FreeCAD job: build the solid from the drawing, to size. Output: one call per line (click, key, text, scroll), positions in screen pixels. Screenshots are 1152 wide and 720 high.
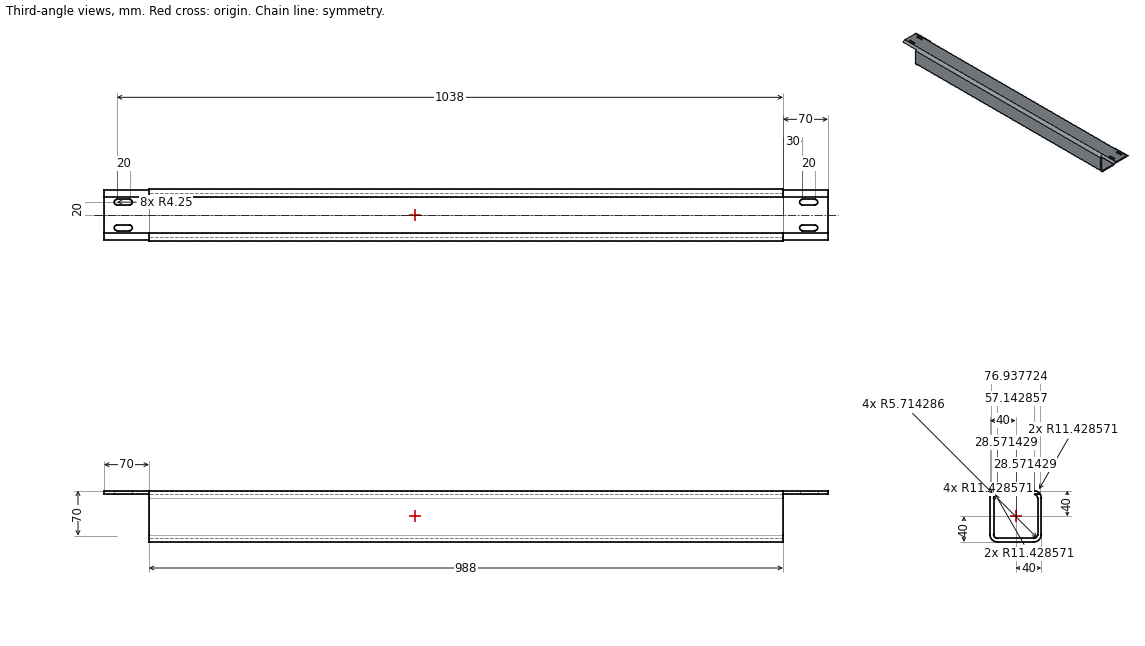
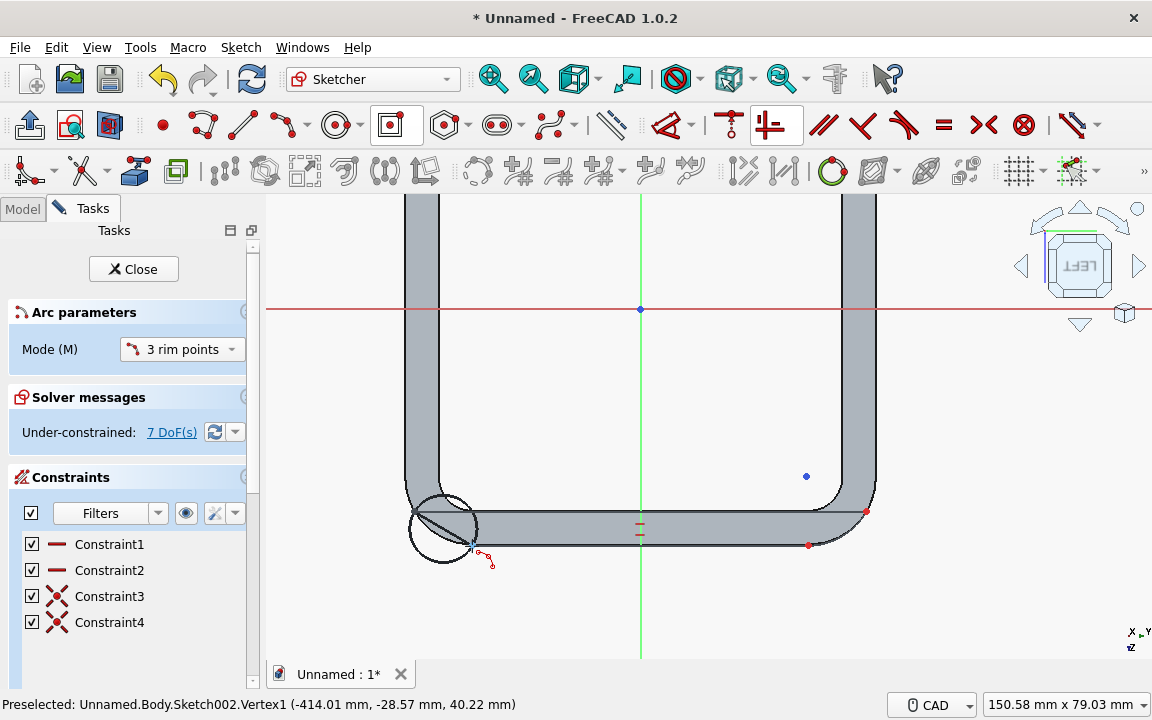
scroll(439, 536, up, 3)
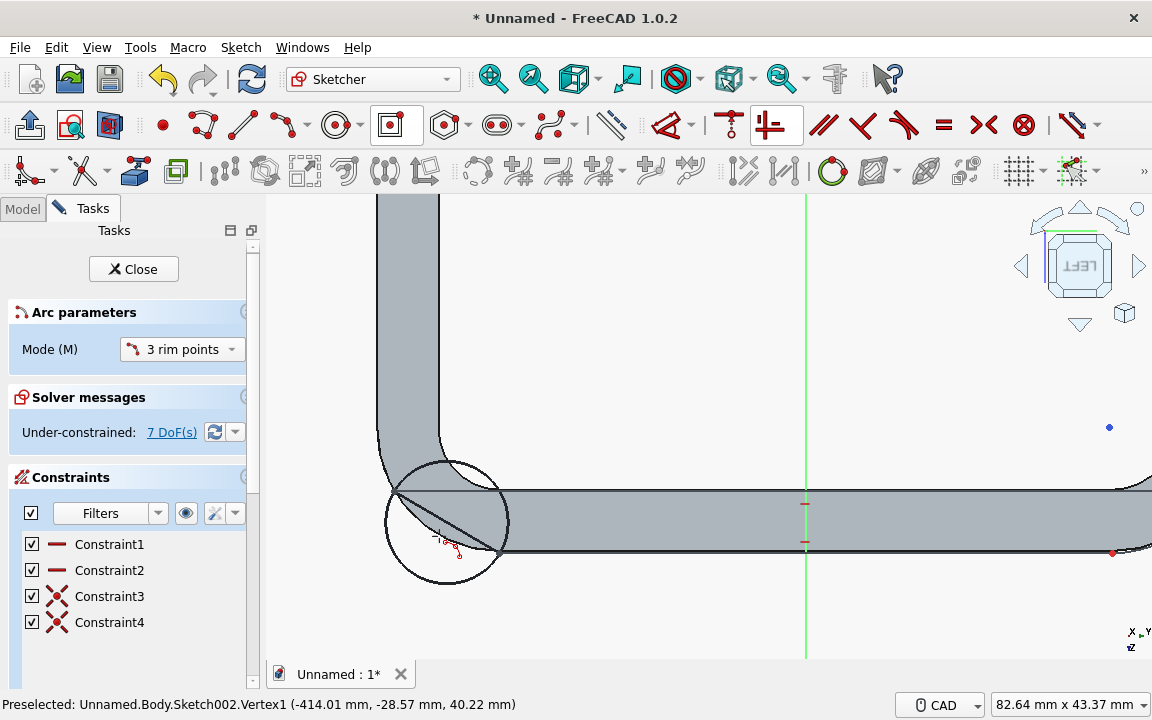
click(439, 535)
key(Escape)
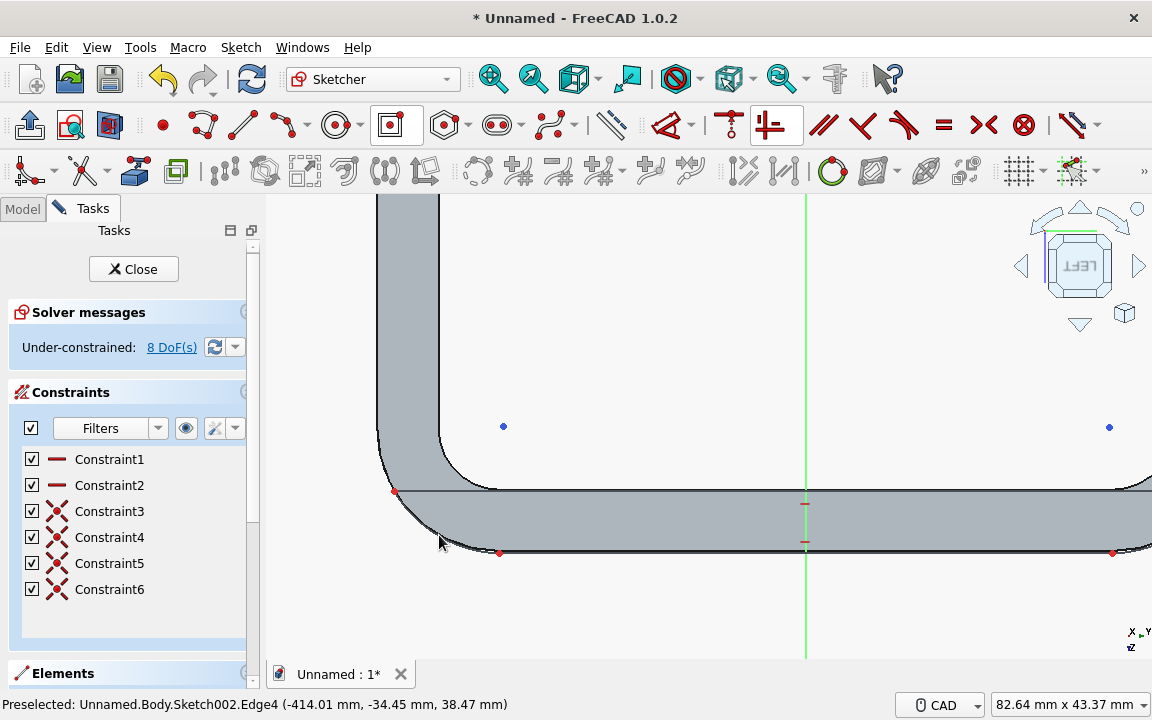
click(683, 553)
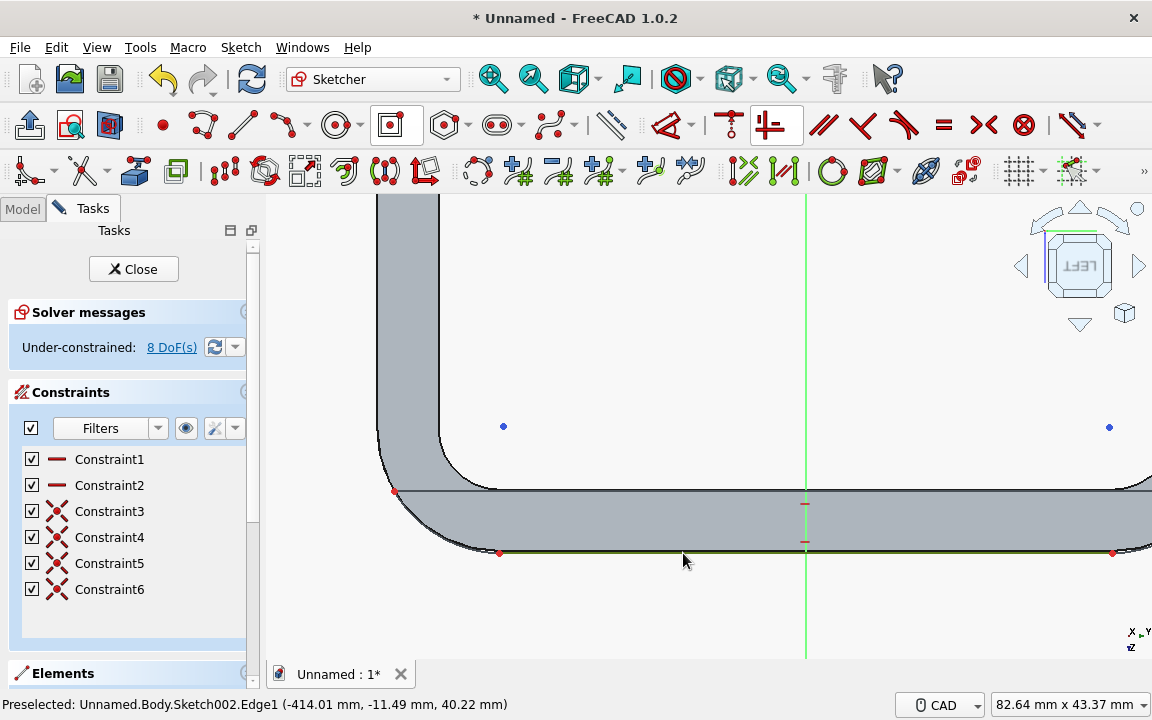
scroll(439, 536, down, 3)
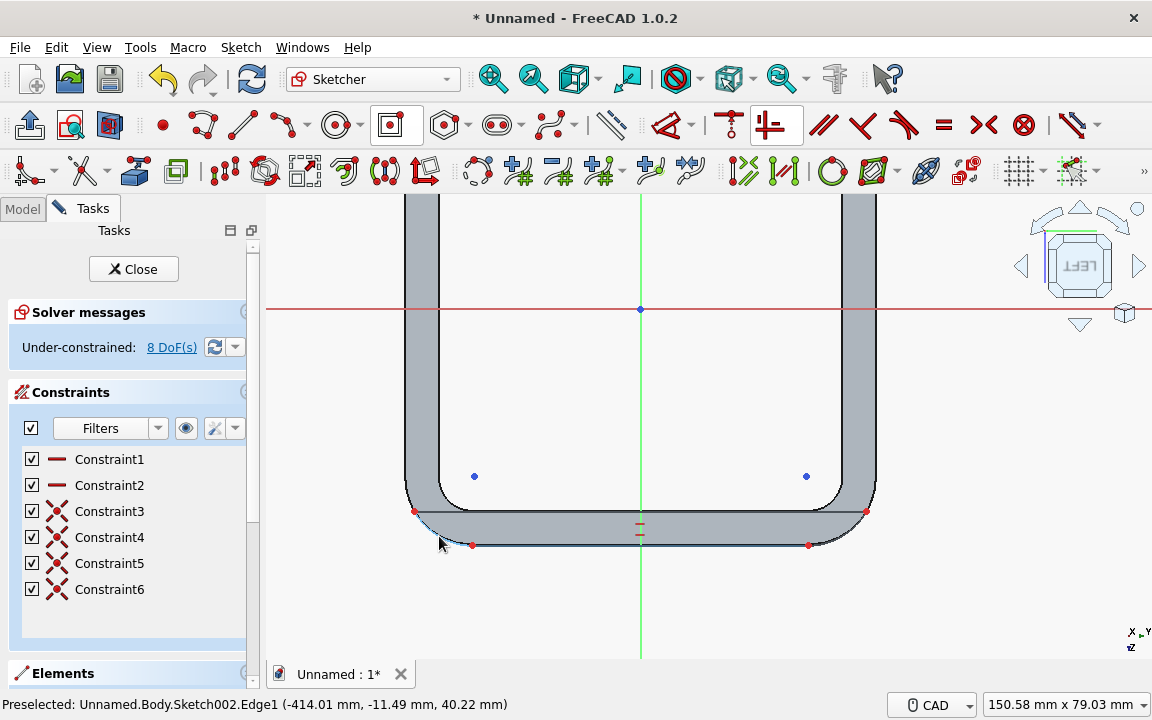
click(829, 542)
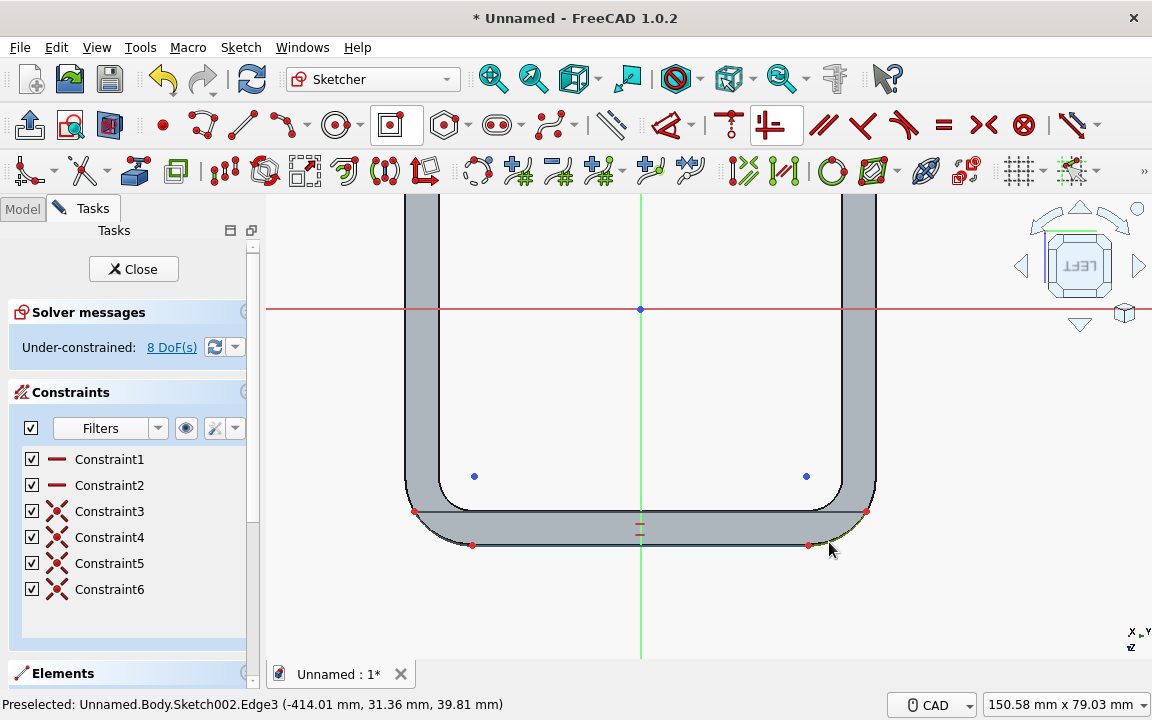
key(t)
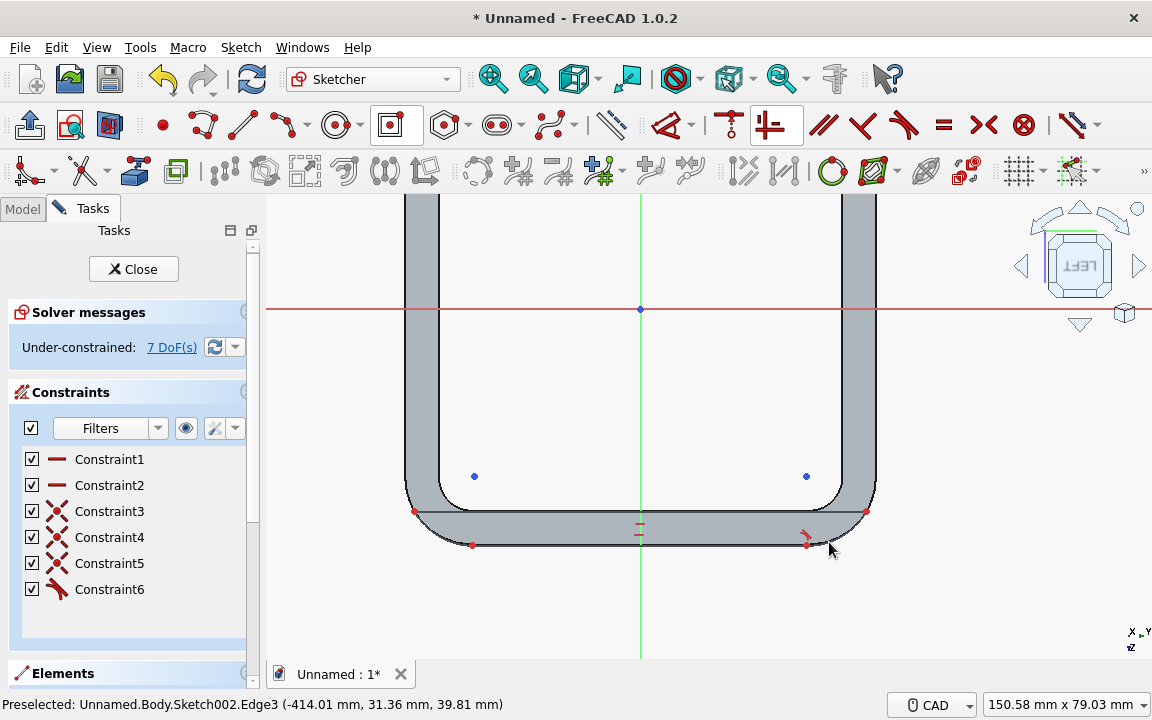
click(573, 546)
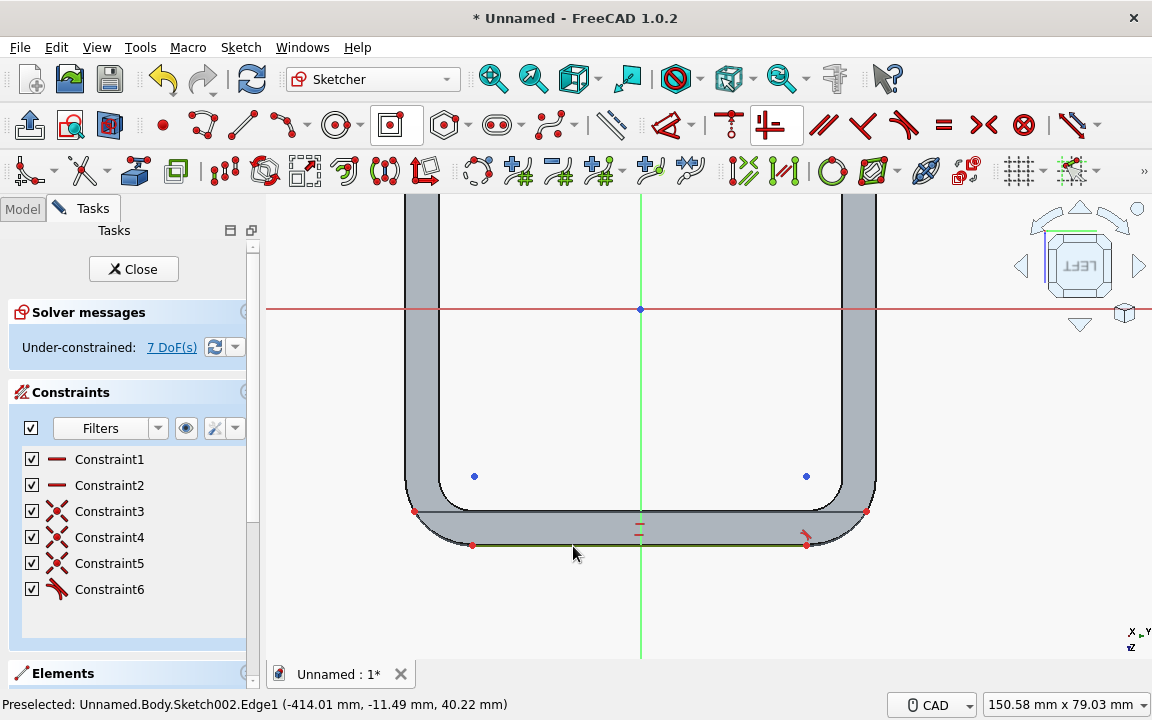
click(428, 528)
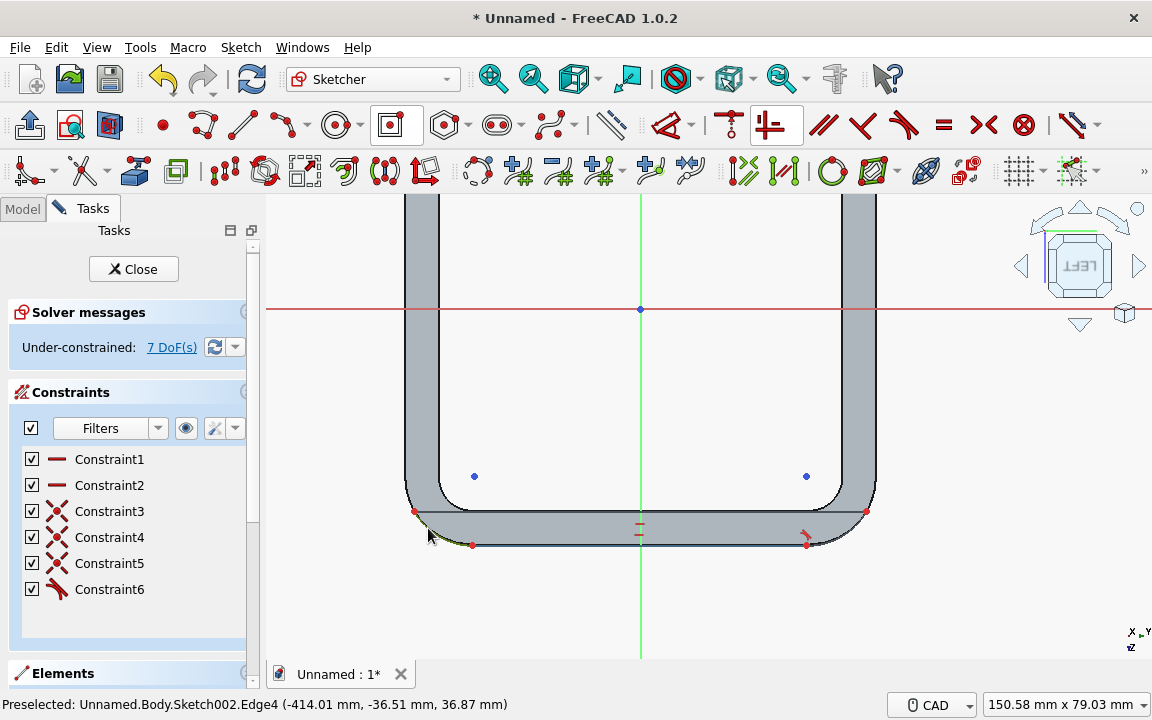
key(t)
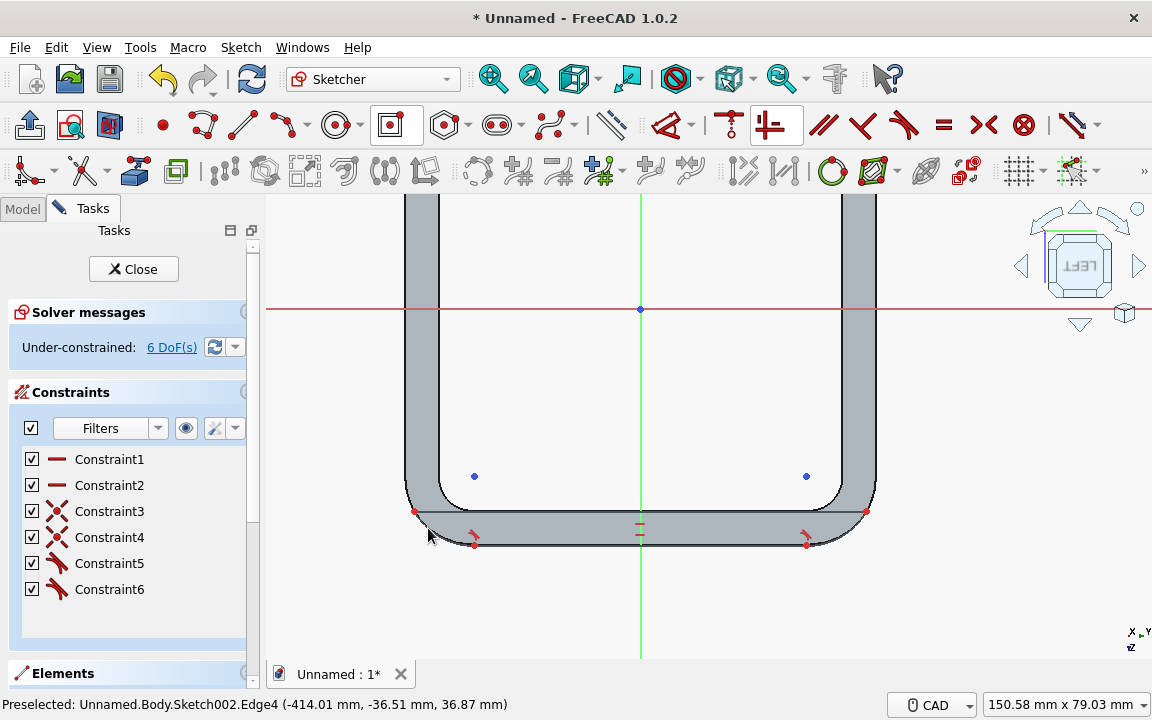
click(828, 543)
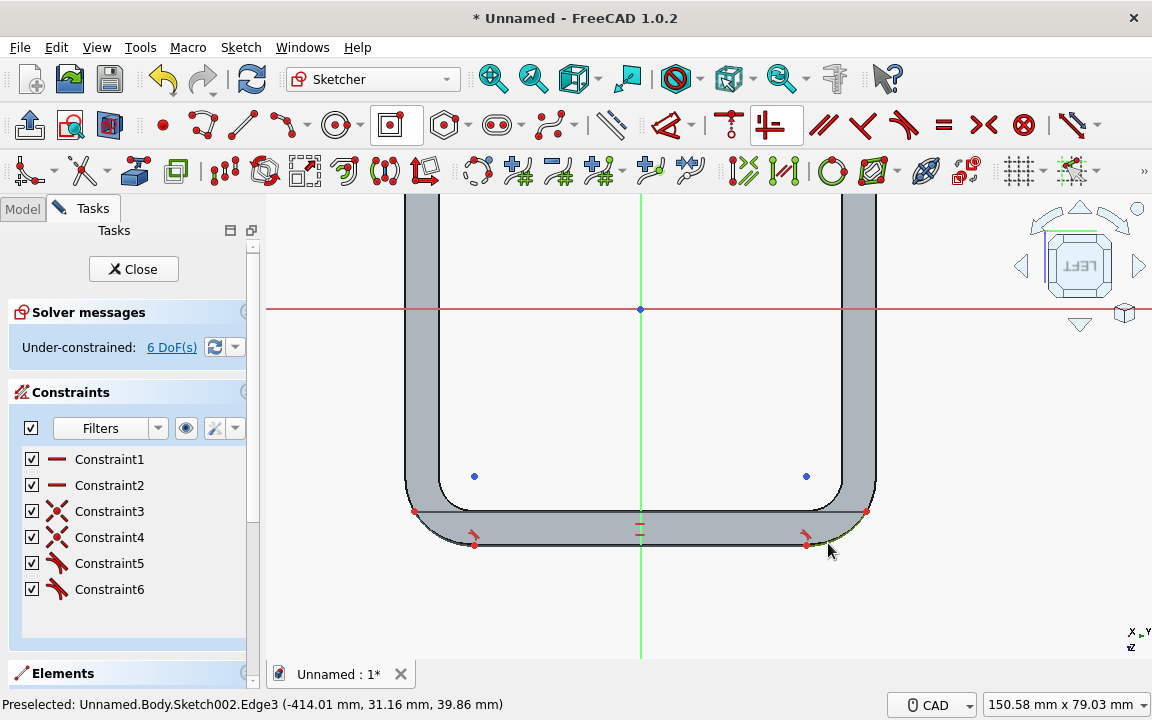
click(428, 528)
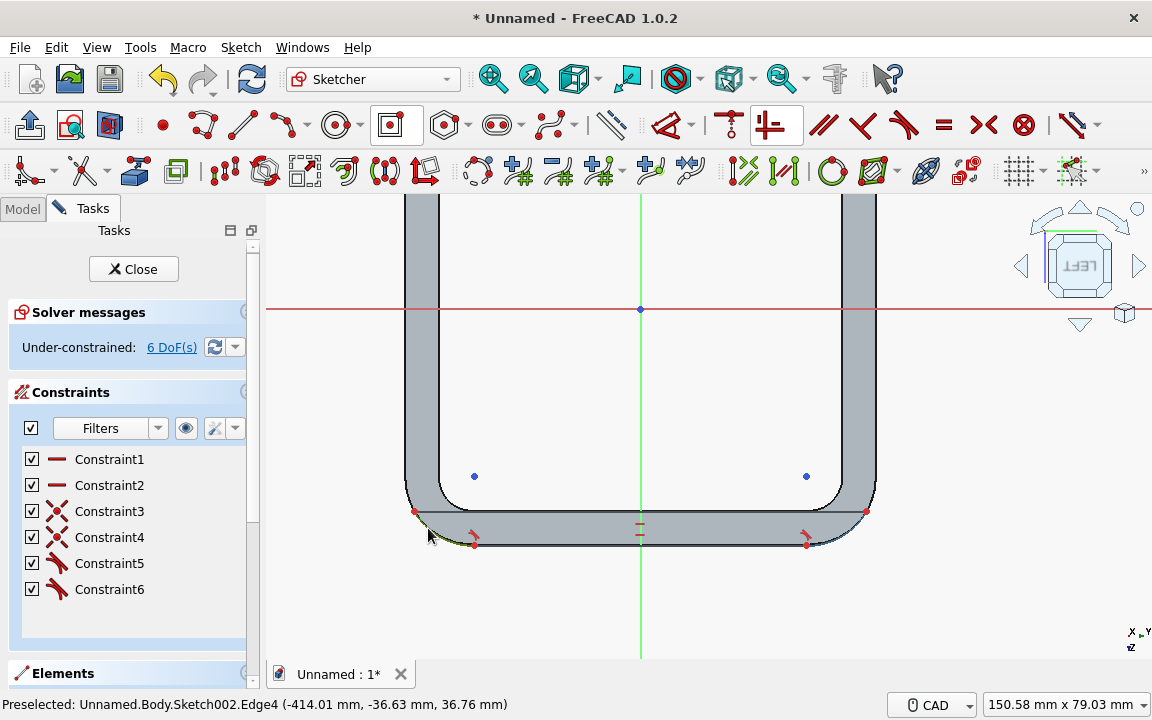
key(e)